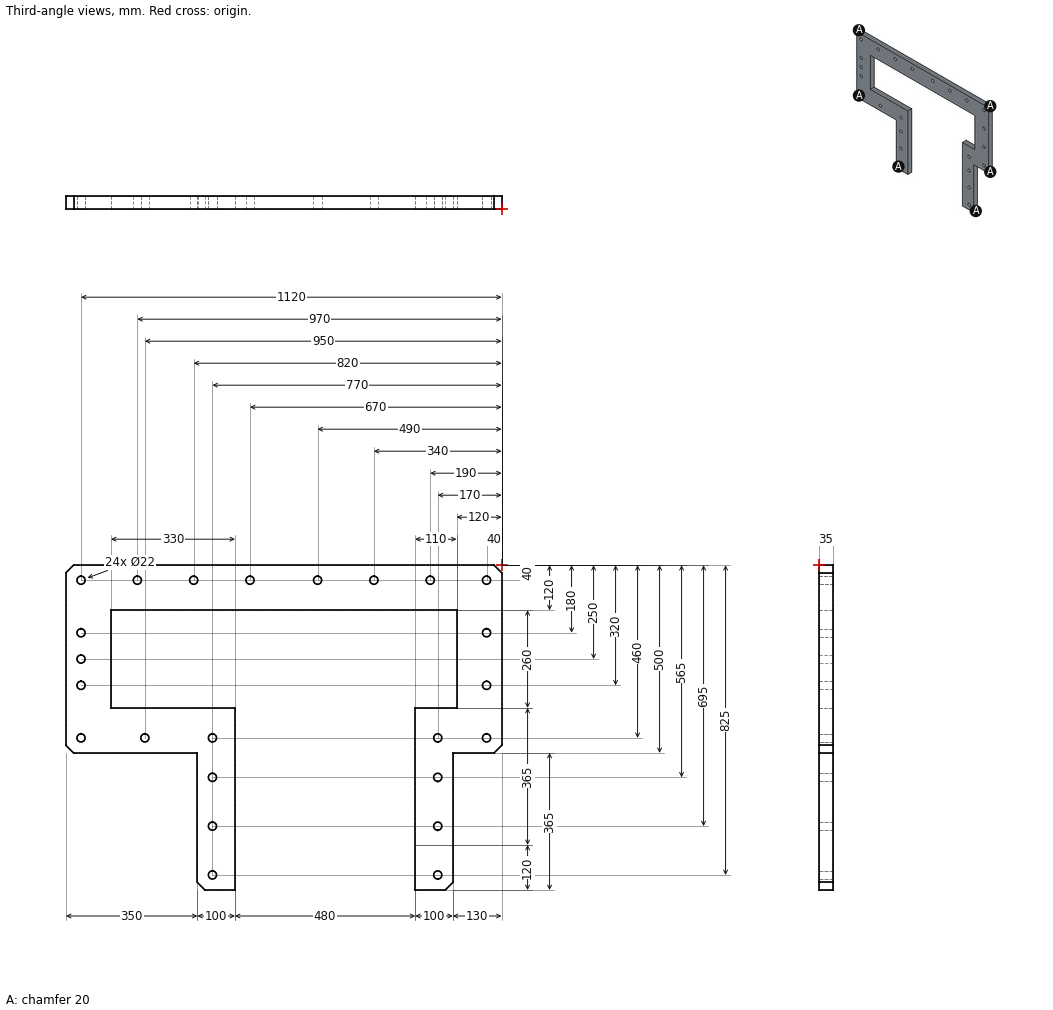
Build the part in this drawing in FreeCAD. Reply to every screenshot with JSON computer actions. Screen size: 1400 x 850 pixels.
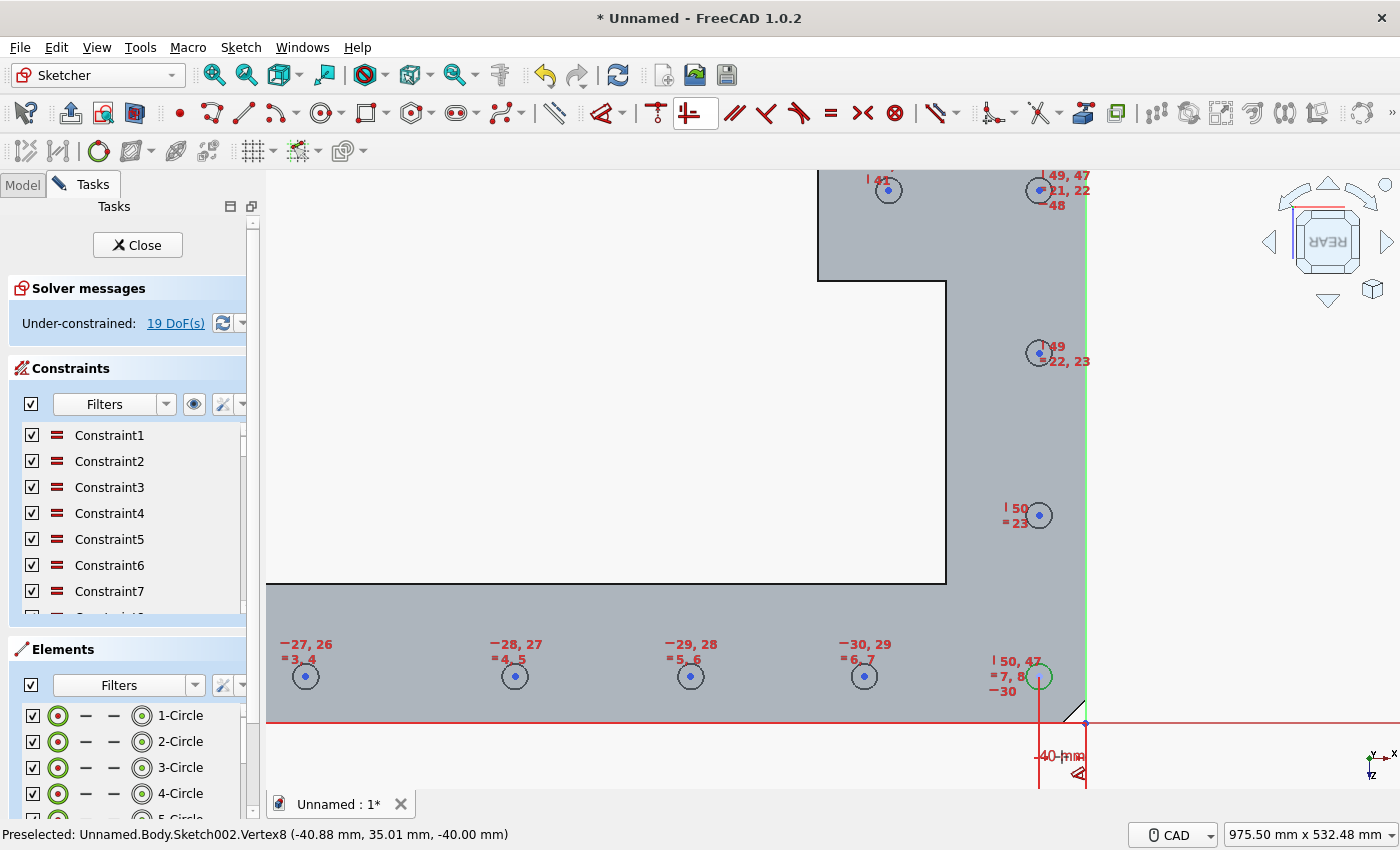
{"action": "scroll", "coordinate": [1039, 677], "scroll_direction": "down", "scroll_amount": 4}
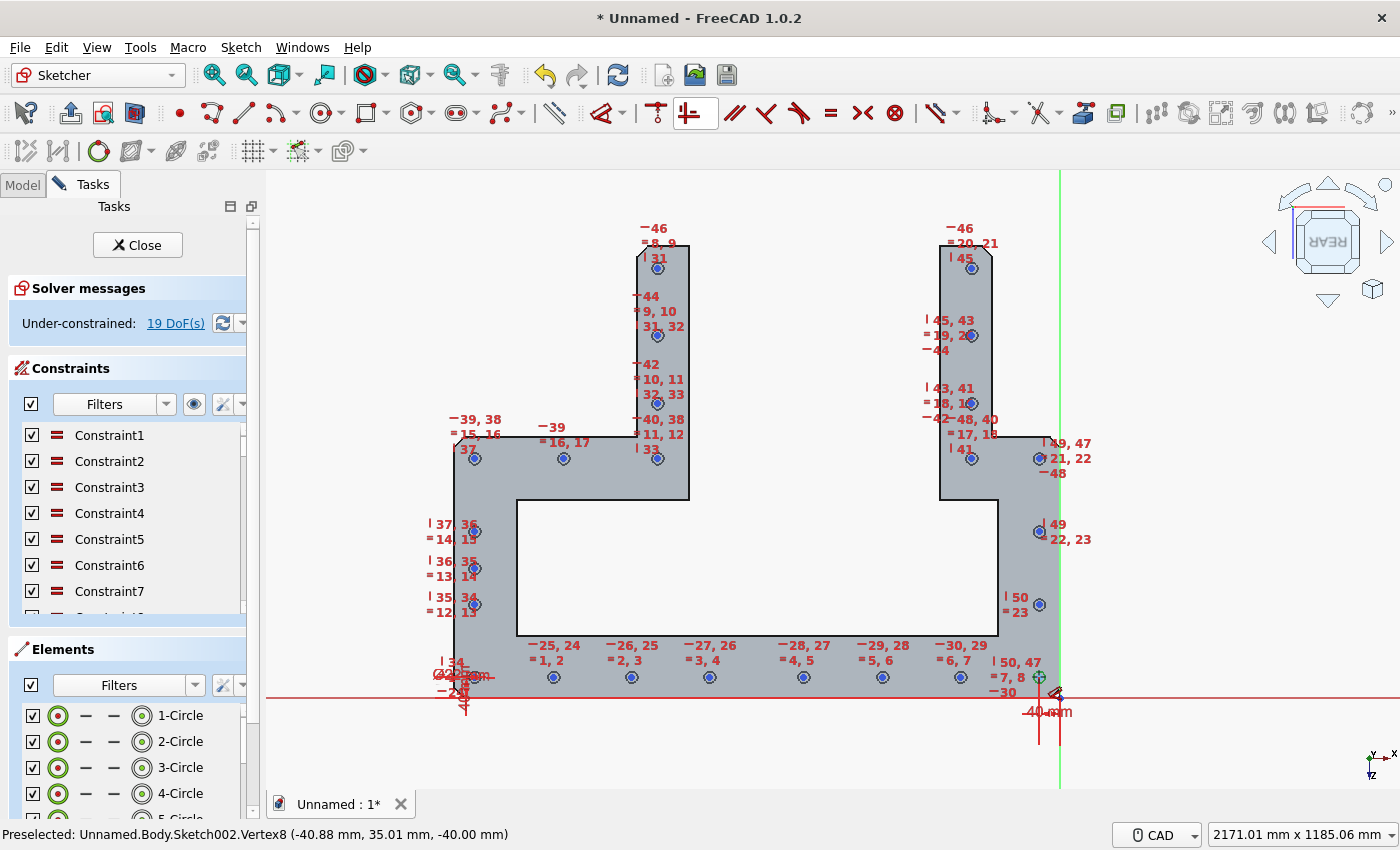
{"action": "left_click", "coordinate": [554, 677]}
{"action": "left_click", "coordinate": [807, 732]}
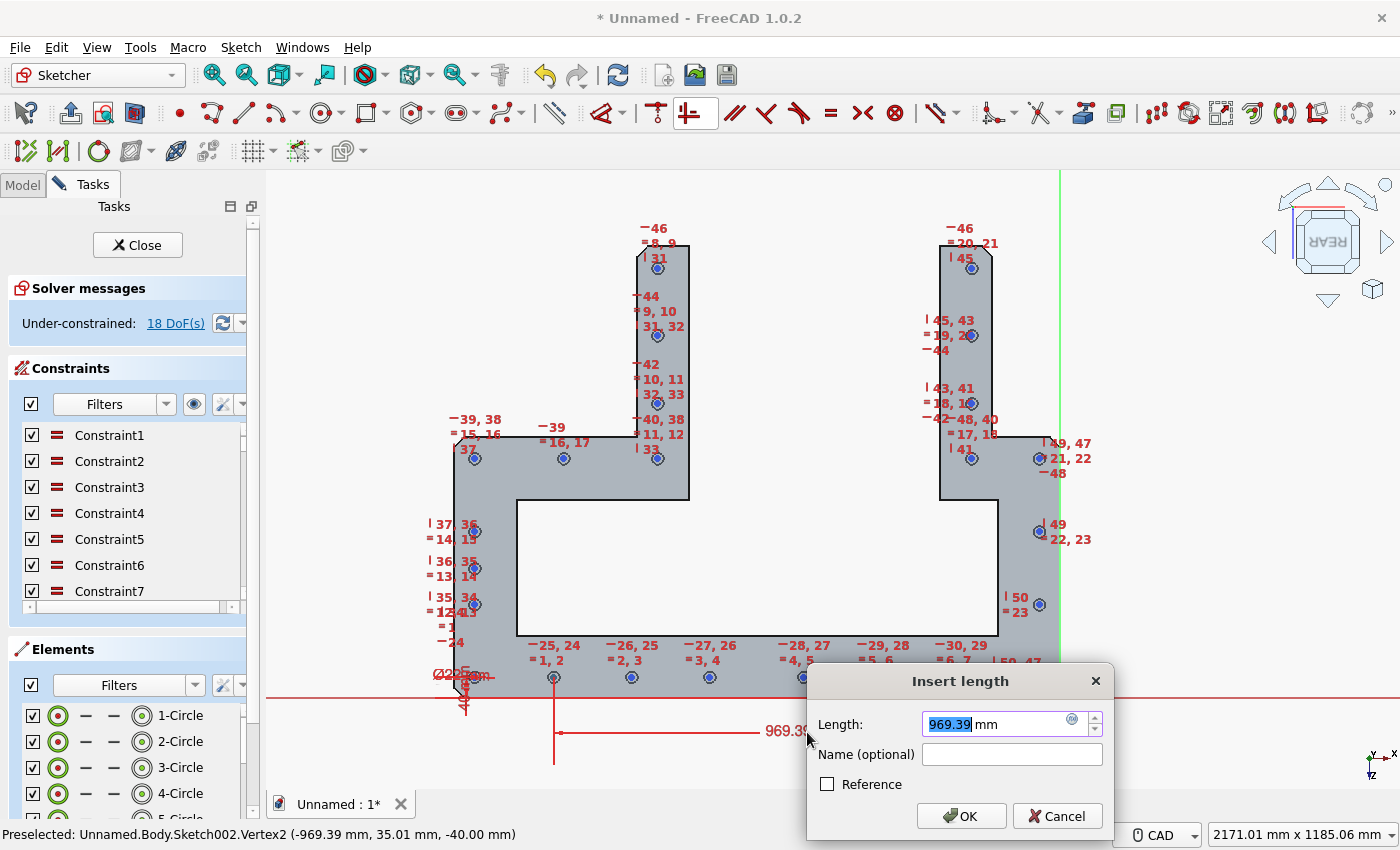
{"action": "type", "text": "970"}
{"action": "key", "text": "Return"}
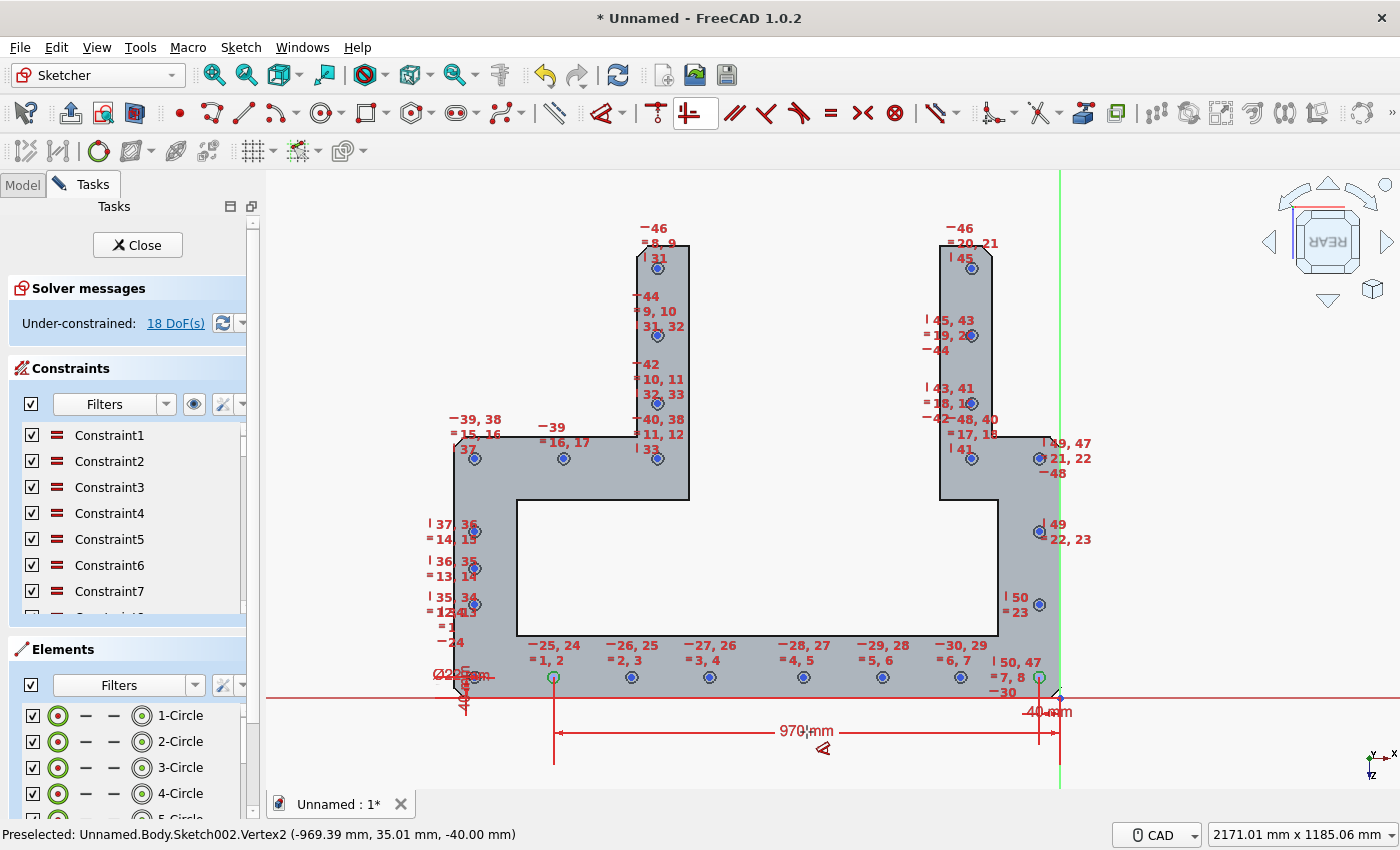
{"action": "left_click", "coordinate": [632, 677]}
{"action": "left_click", "coordinate": [945, 732]}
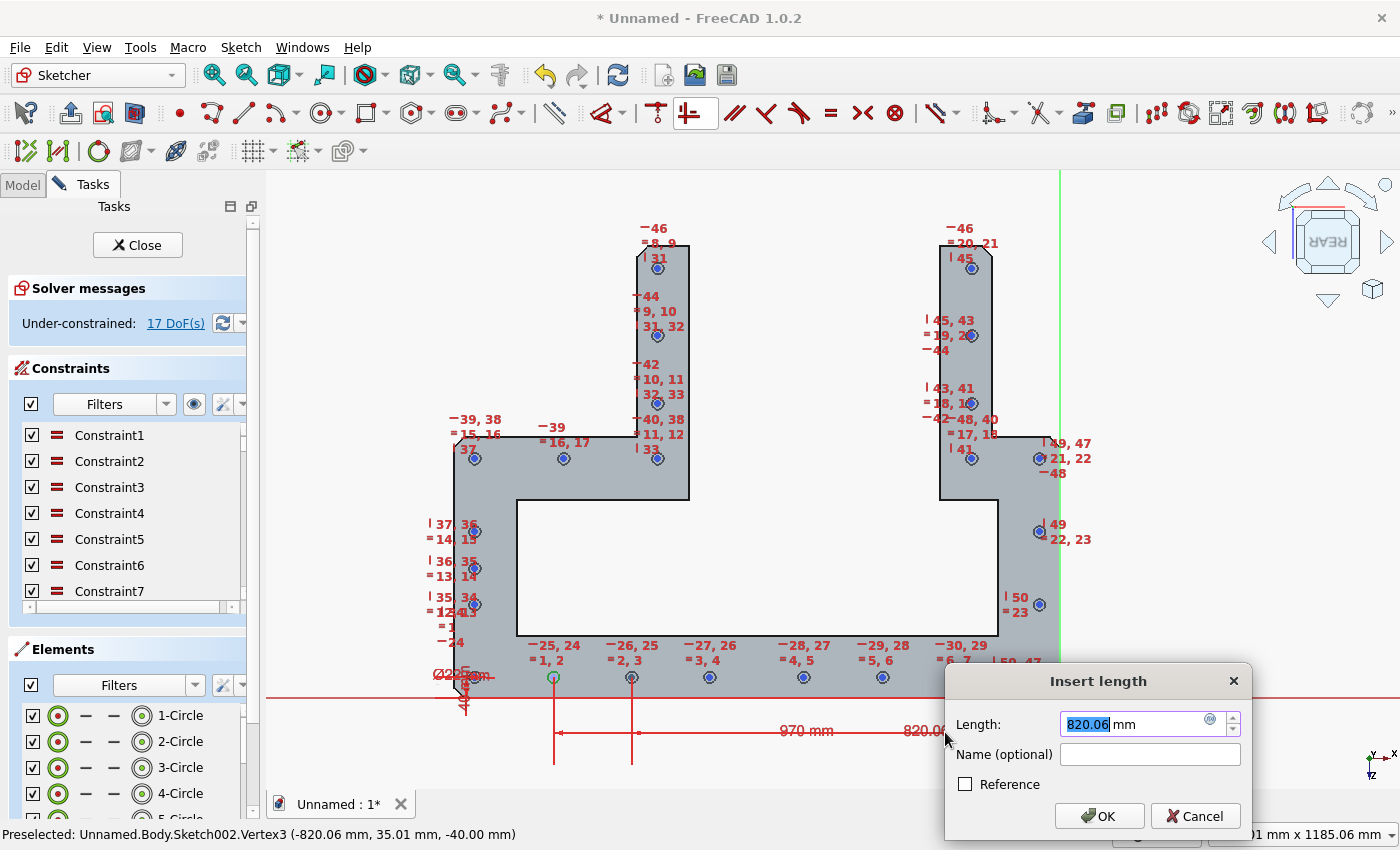
{"action": "type", "text": "820"}
{"action": "key", "text": "Return"}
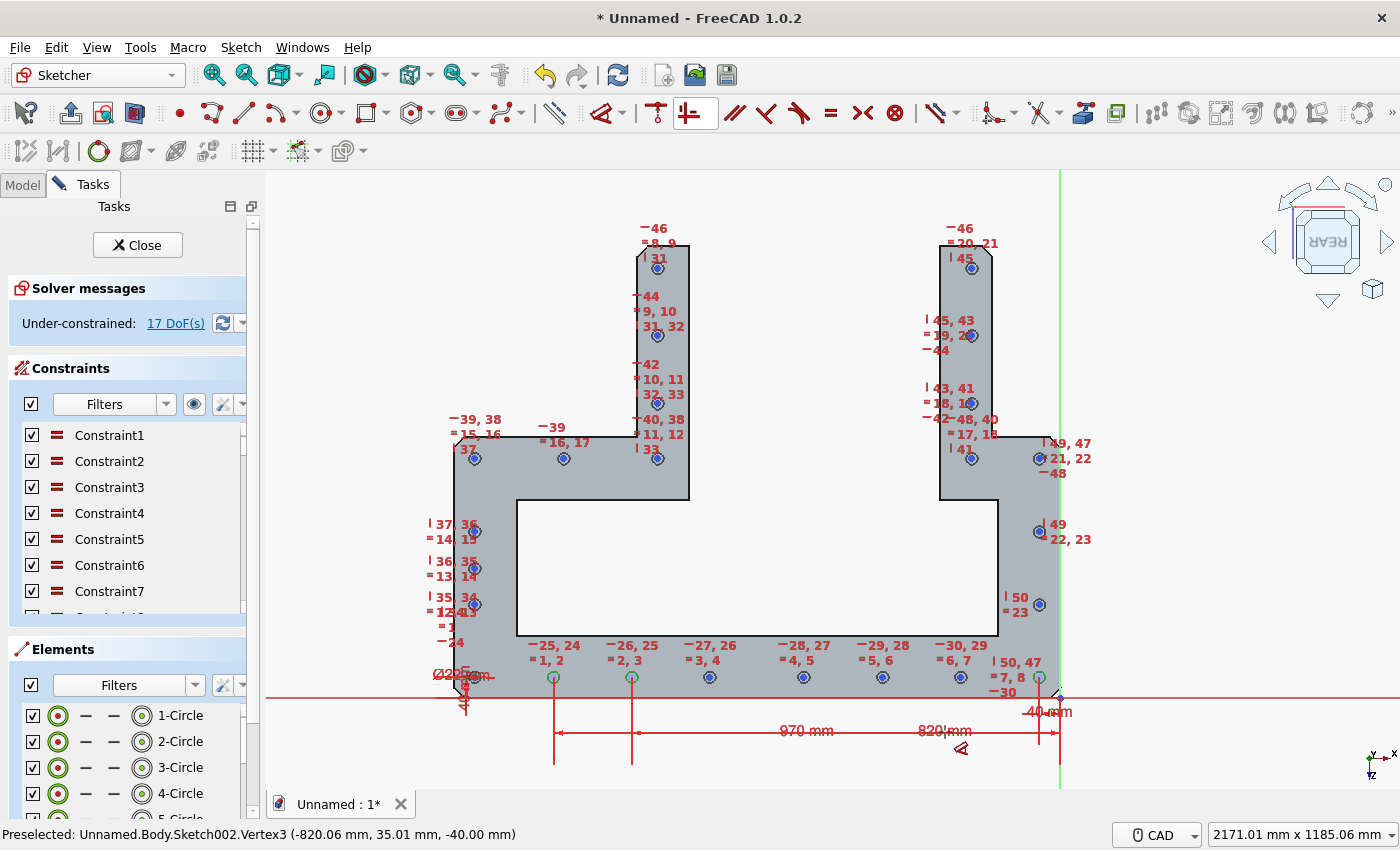
{"action": "left_click", "coordinate": [710, 677]}
{"action": "left_click", "coordinate": [885, 643]}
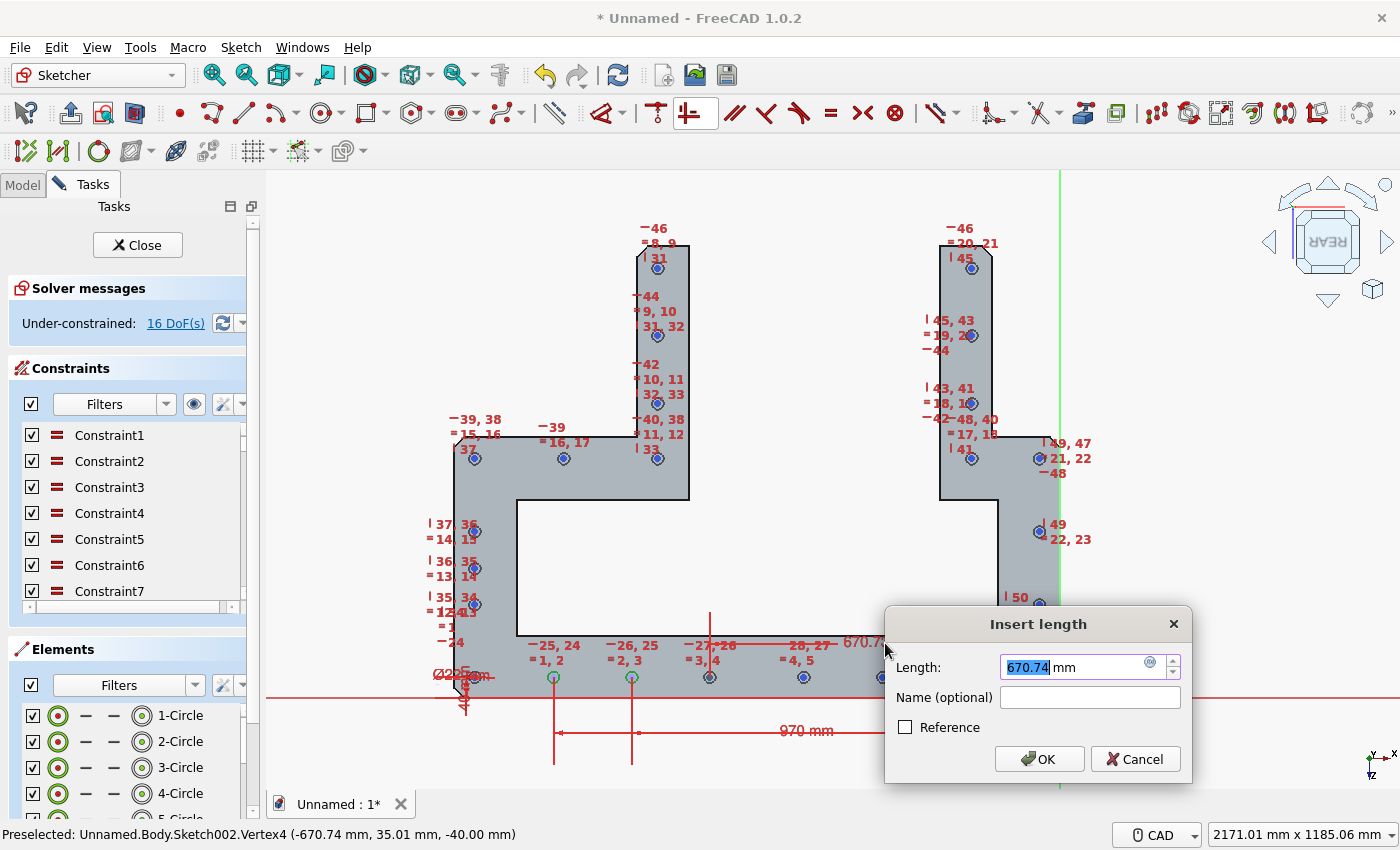
{"action": "type", "text": "670"}
{"action": "key", "text": "Return"}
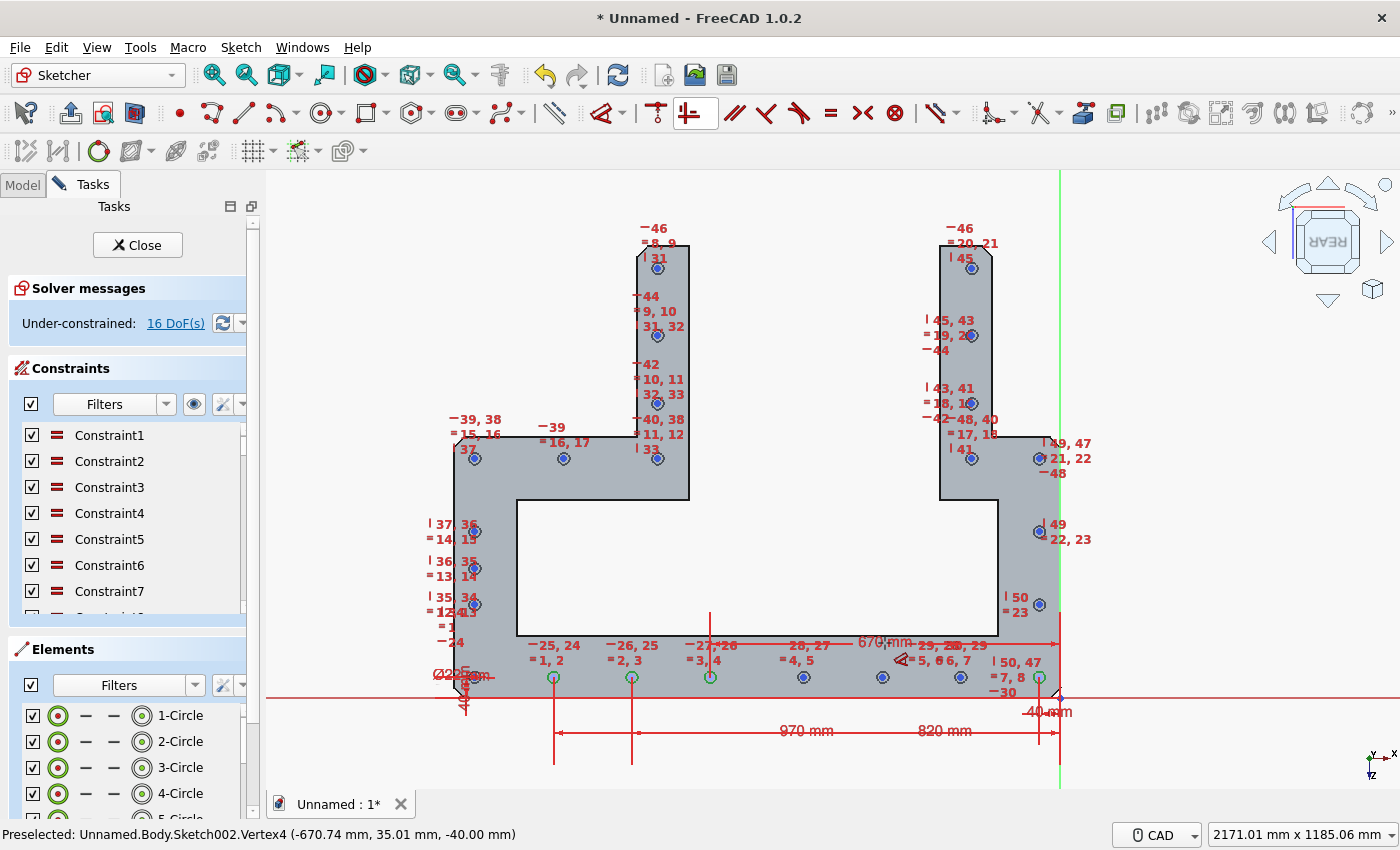
{"action": "left_click", "coordinate": [804, 677]}
{"action": "left_click", "coordinate": [991, 643]}